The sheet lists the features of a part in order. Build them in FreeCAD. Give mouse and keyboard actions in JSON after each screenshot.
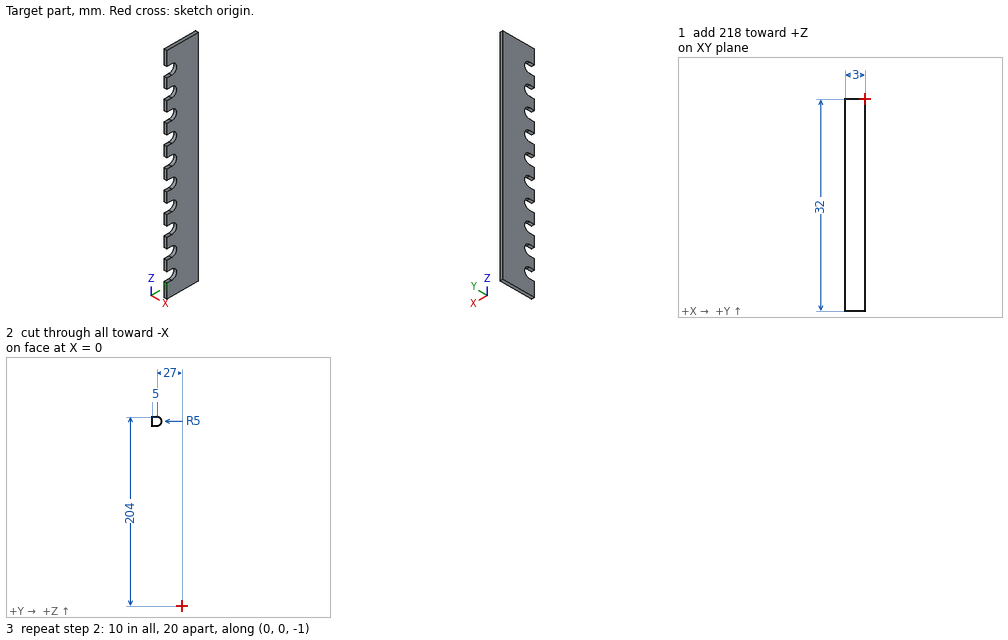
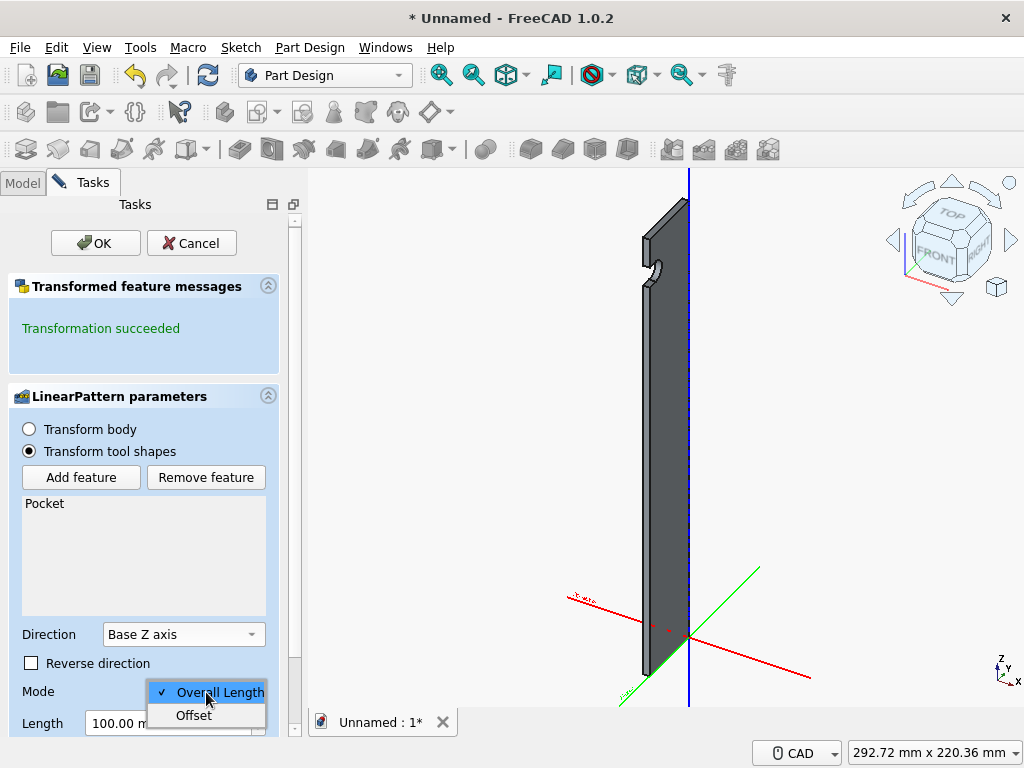
{"action": "left_click", "coordinate": [206, 716]}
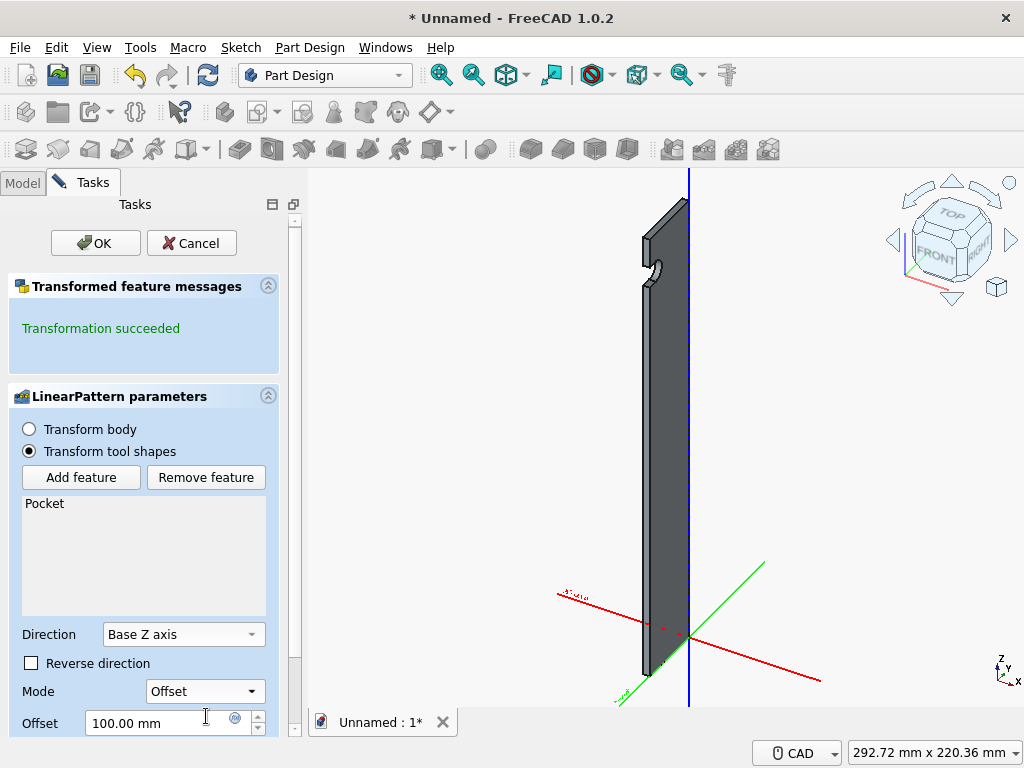
{"action": "triple_click", "coordinate": [168, 723]}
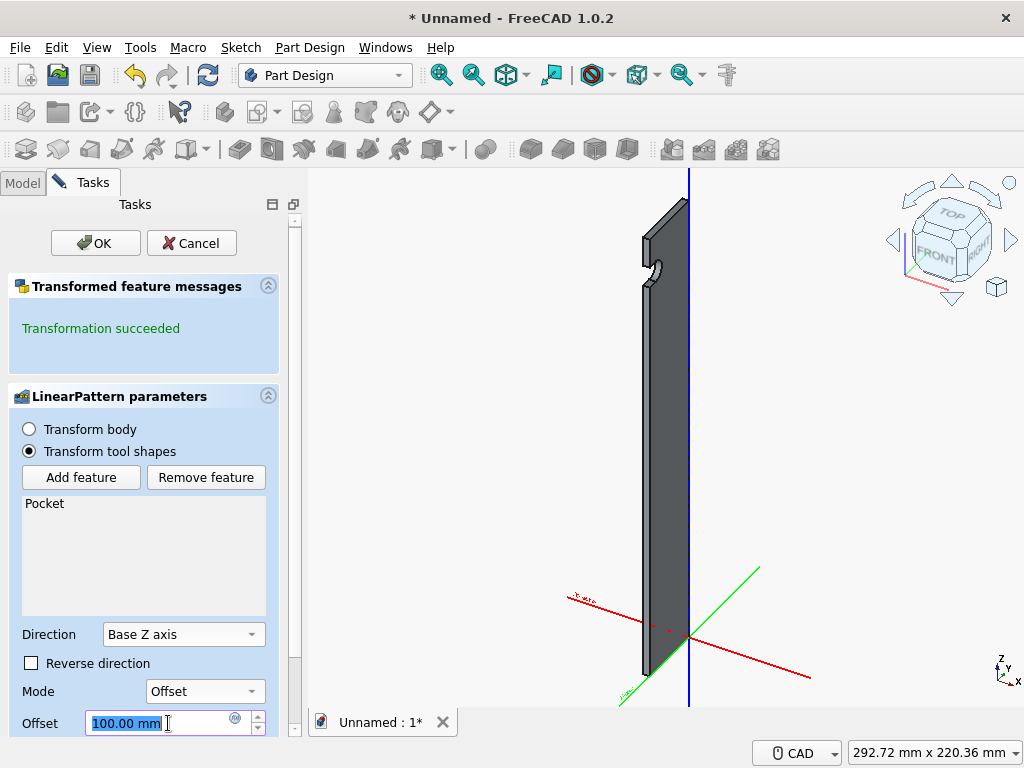
{"action": "type", "text": "20"}
{"action": "key", "text": "Tab"}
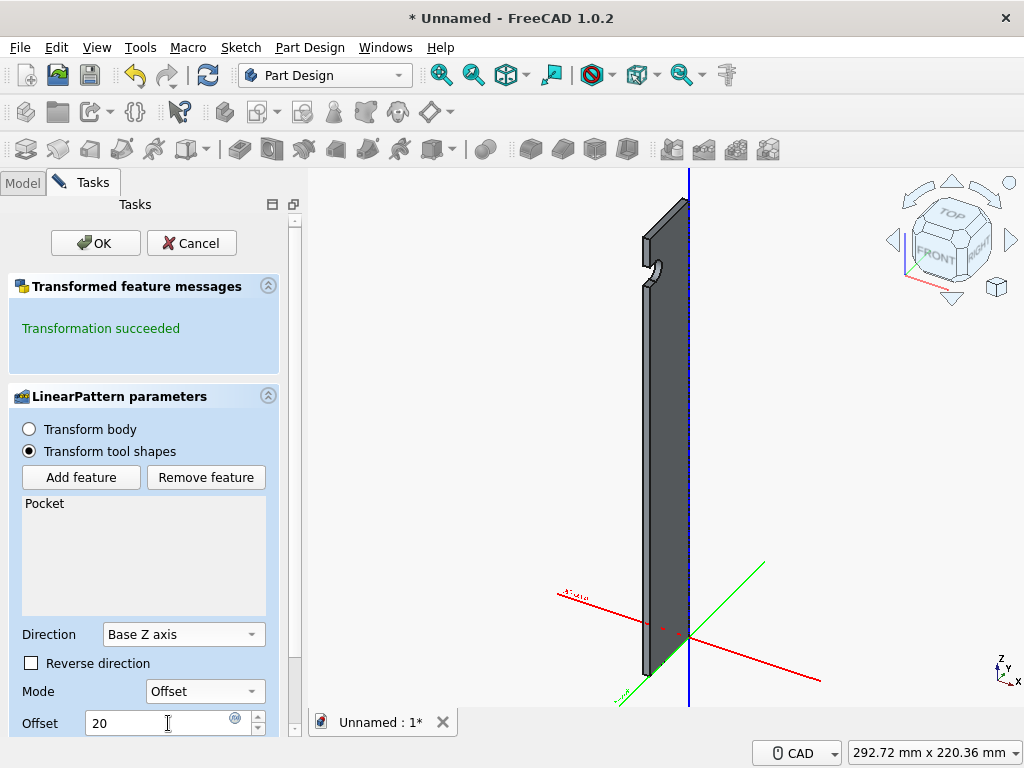
{"action": "scroll", "coordinate": [295, 475], "scroll_direction": "down", "scroll_amount": 2}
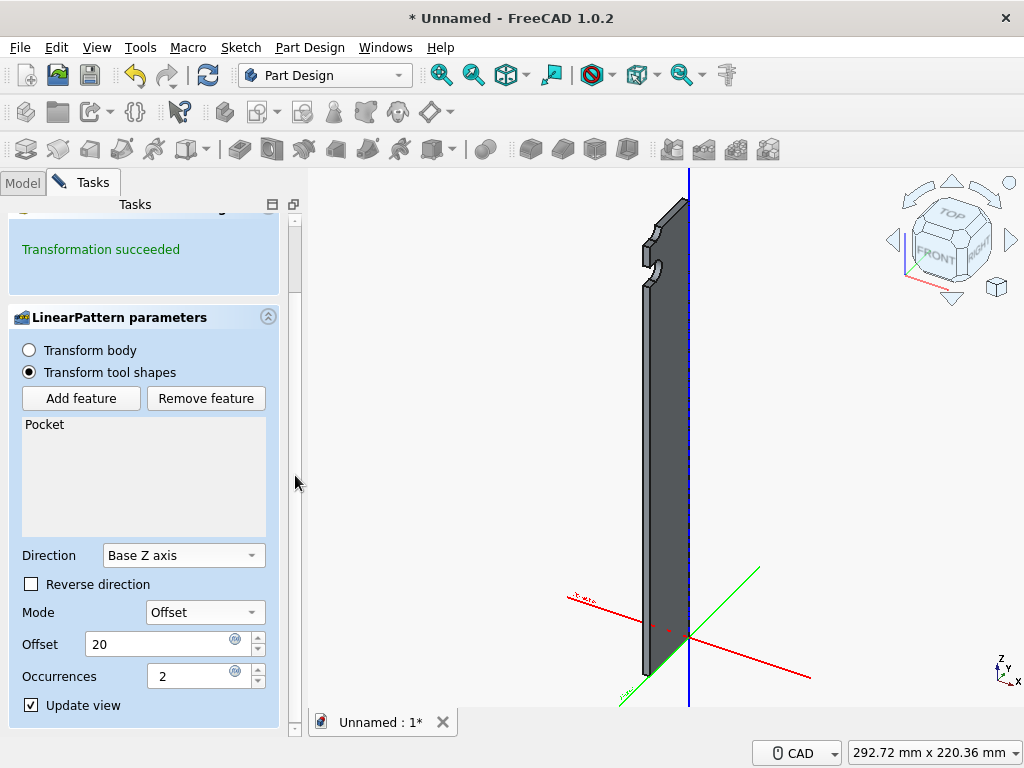
{"action": "triple_click", "coordinate": [198, 676]}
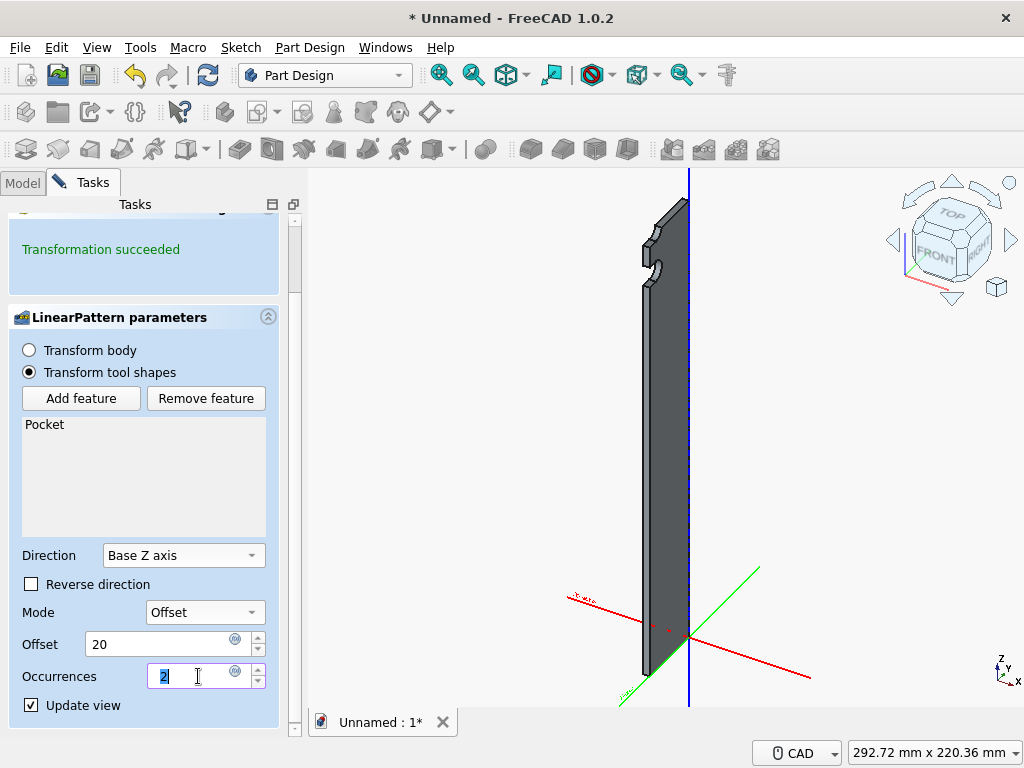
{"action": "type", "text": "10"}
{"action": "key", "text": "Tab"}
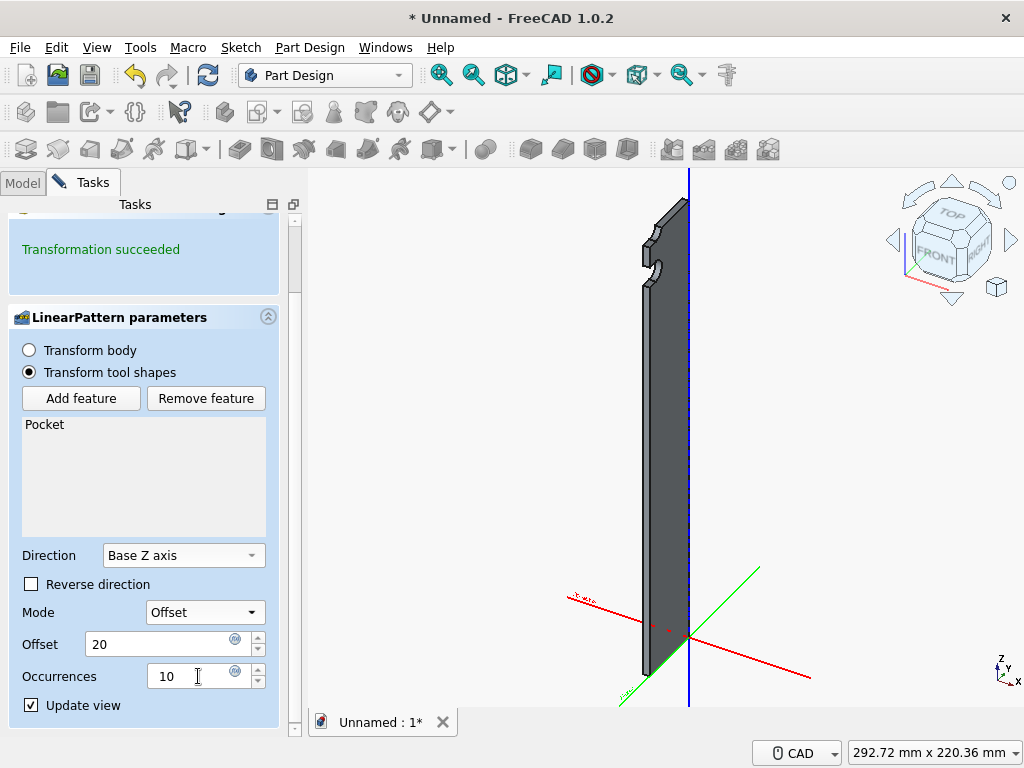
{"action": "left_click", "coordinate": [30, 584]}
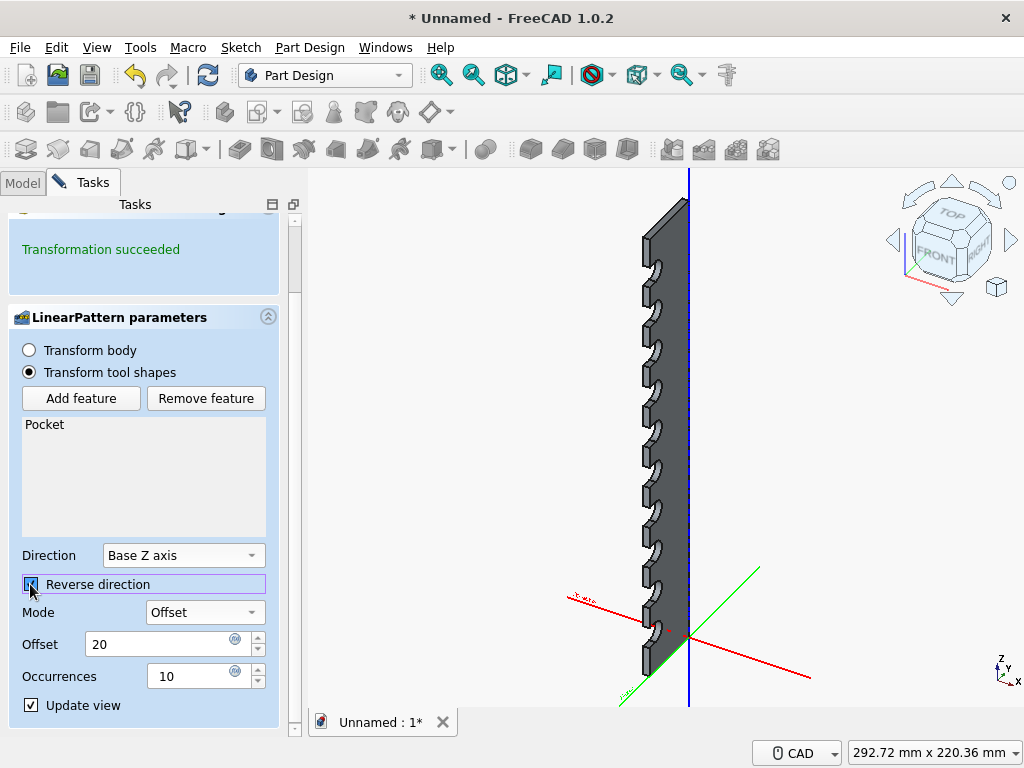
{"action": "scroll", "coordinate": [295, 475], "scroll_direction": "up", "scroll_amount": 3}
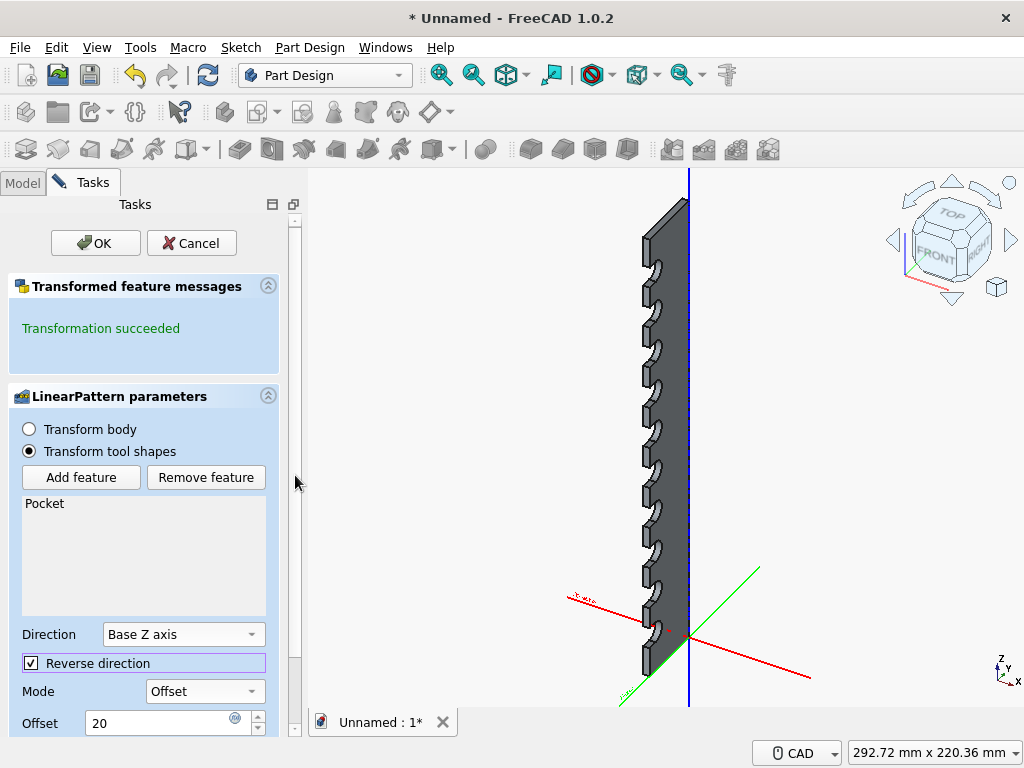
{"action": "left_click", "coordinate": [96, 243]}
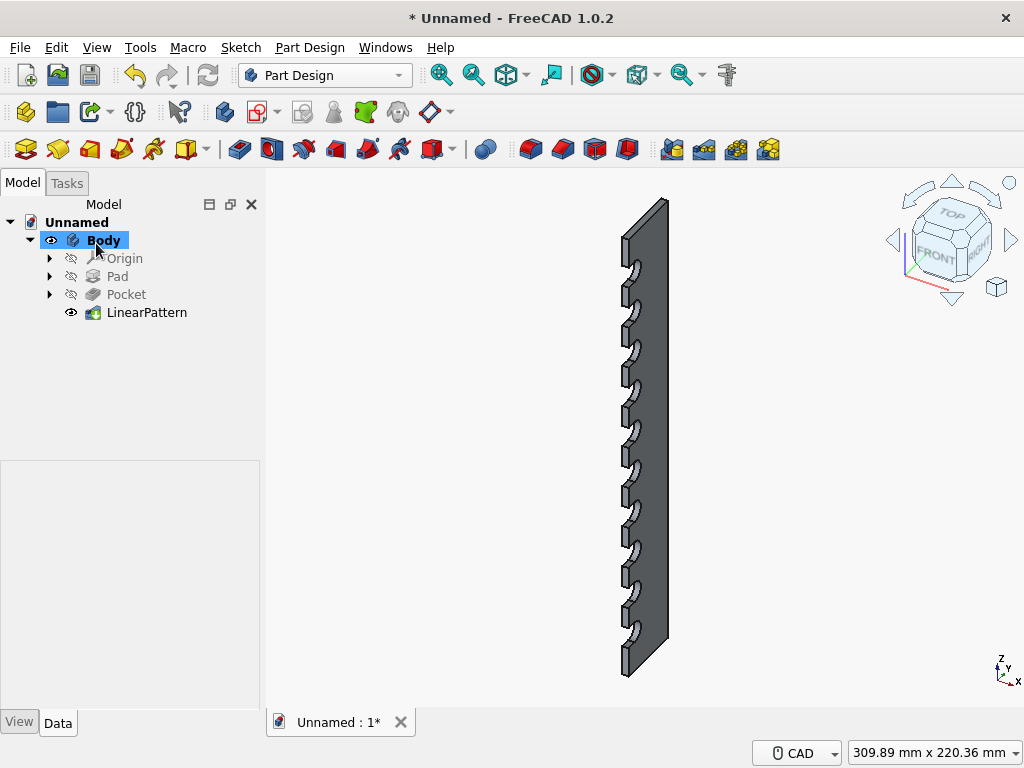
{"action": "key", "text": "0"}